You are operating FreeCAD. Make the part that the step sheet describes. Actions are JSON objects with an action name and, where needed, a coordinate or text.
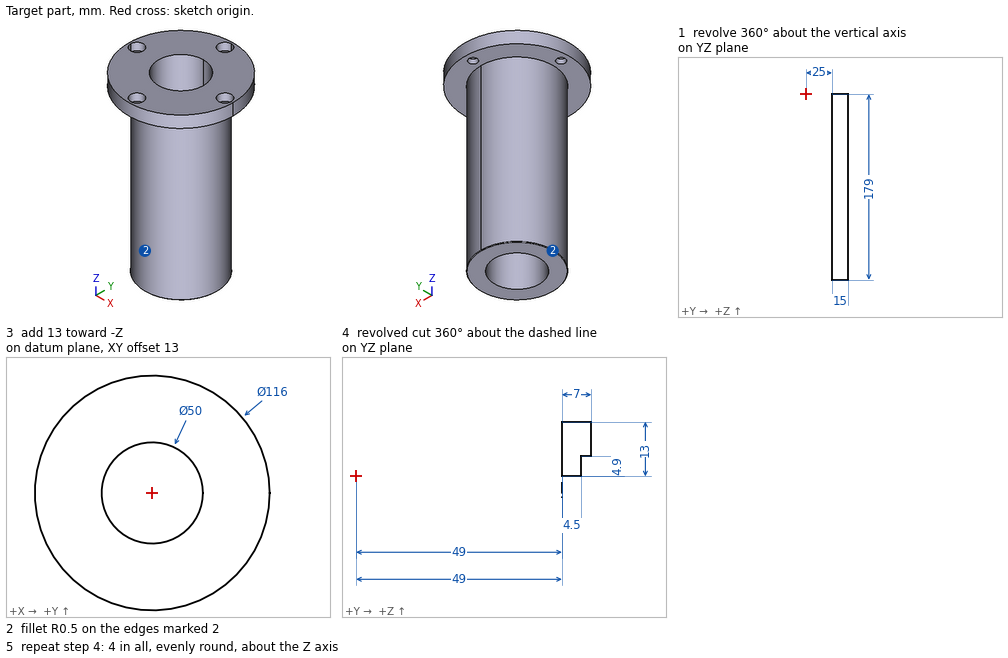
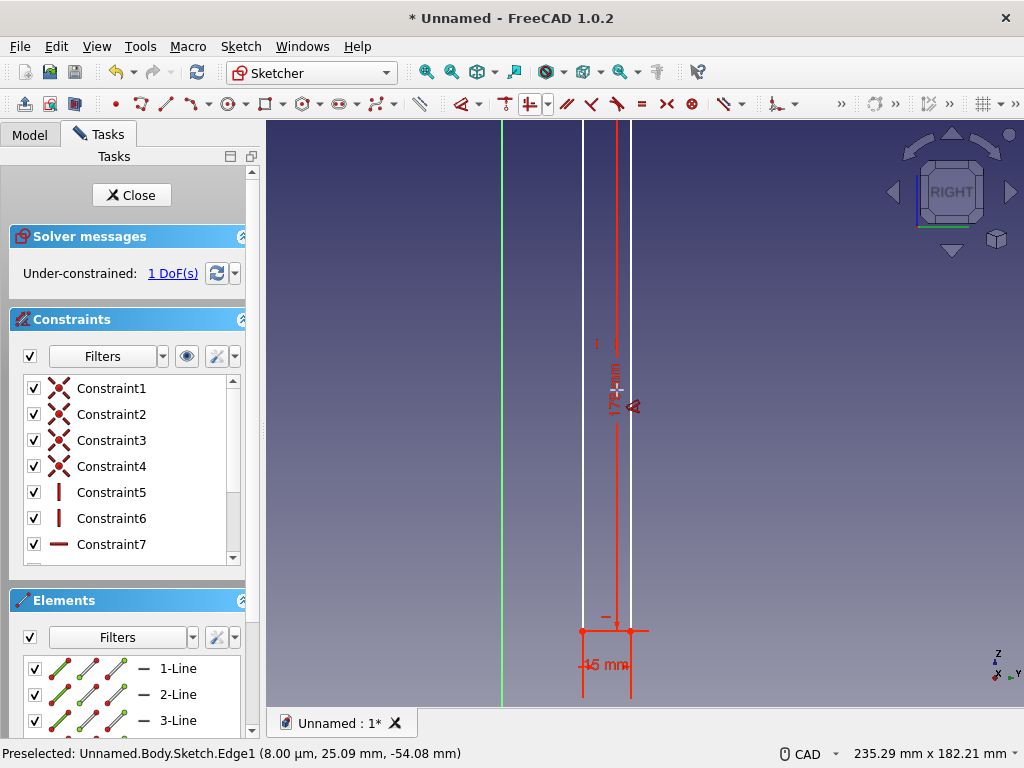
{"action": "scroll", "coordinate": [598, 557], "scroll_direction": "down", "scroll_amount": 2}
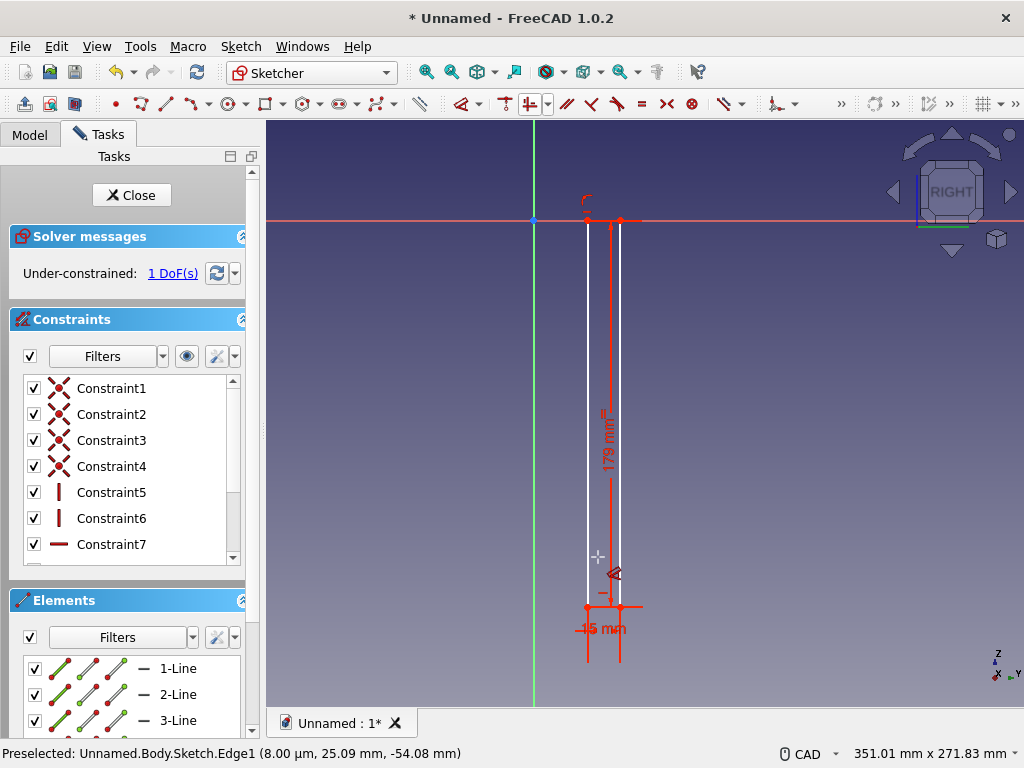
{"action": "left_click", "coordinate": [588, 221]}
{"action": "left_click", "coordinate": [561, 187]}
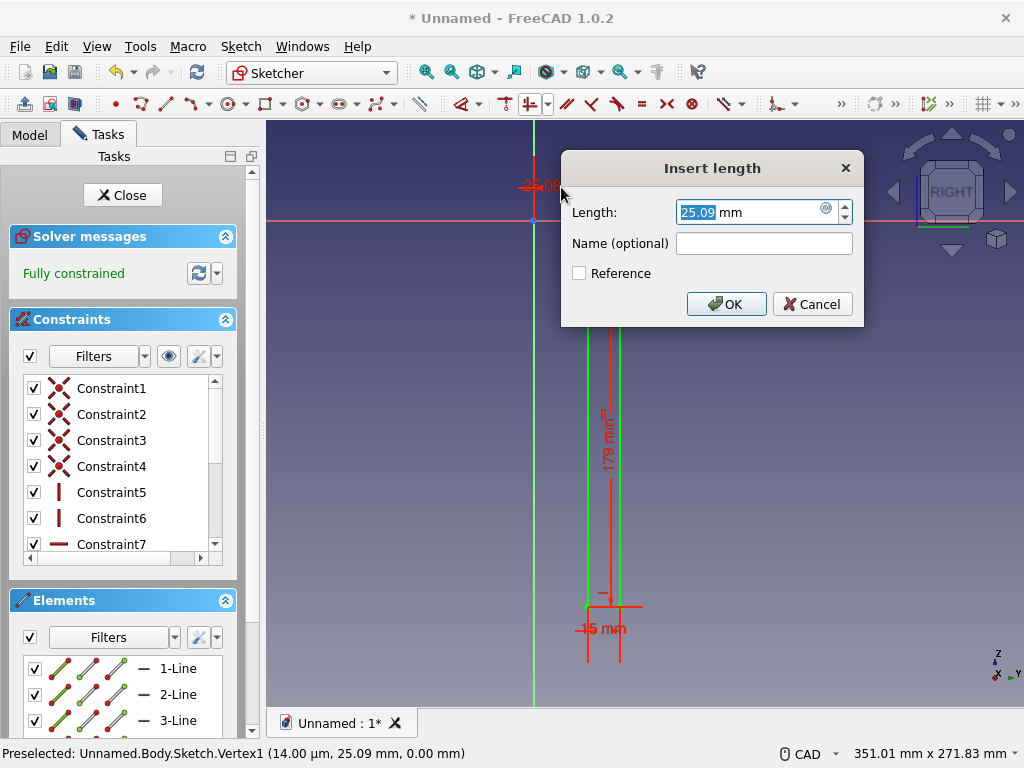
{"action": "type", "text": "25"}
{"action": "key", "text": "Return"}
{"action": "key", "text": "Escape"}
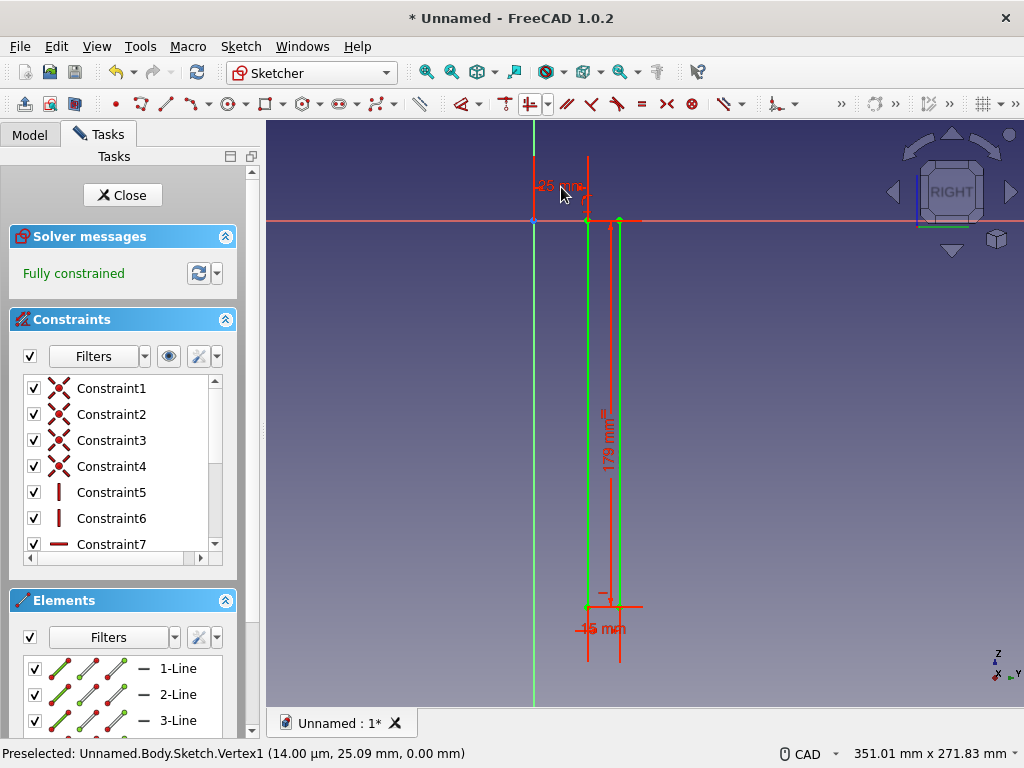
{"action": "left_click", "coordinate": [123, 195]}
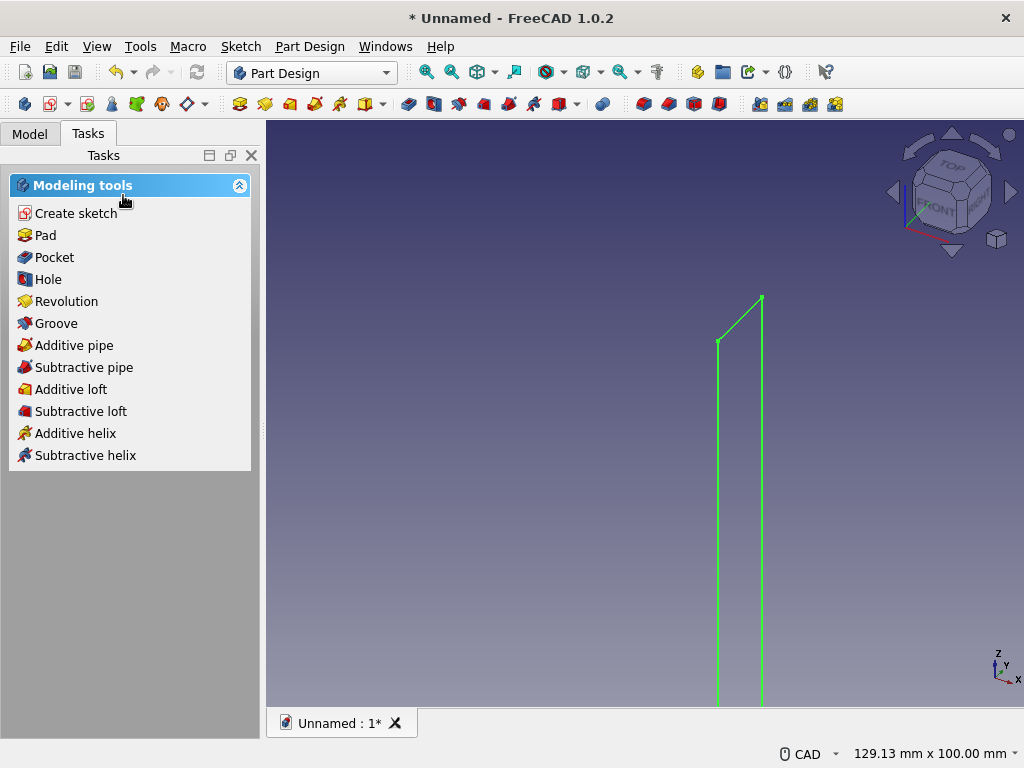
{"action": "left_click", "coordinate": [265, 104]}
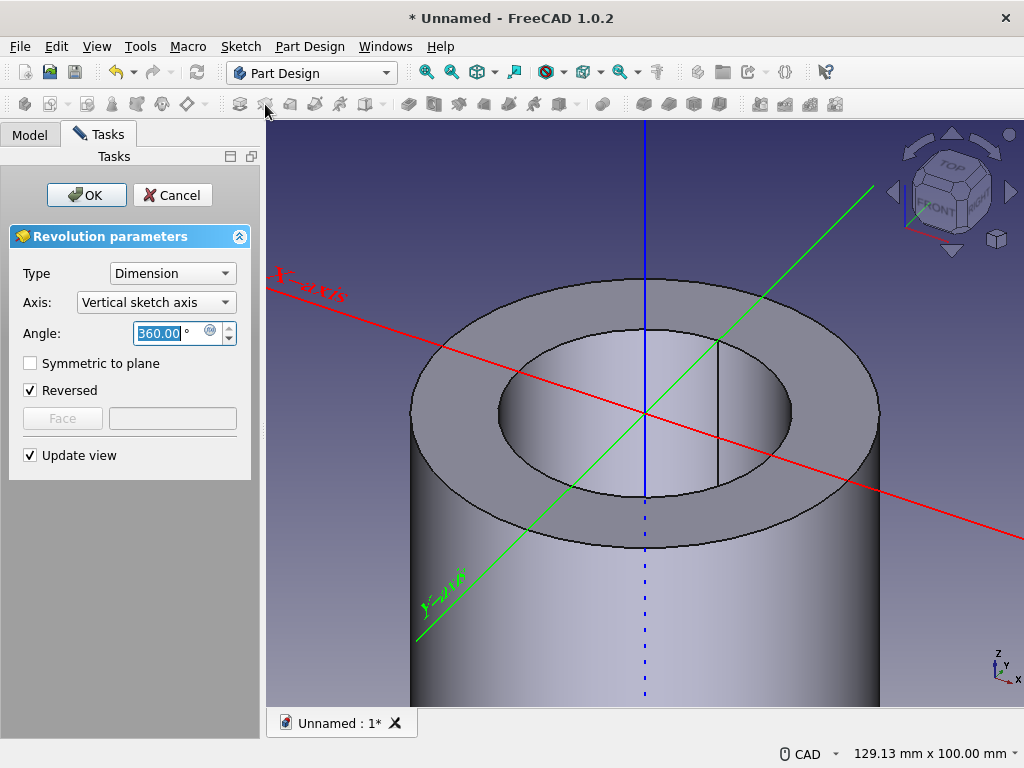
{"action": "left_click", "coordinate": [87, 195]}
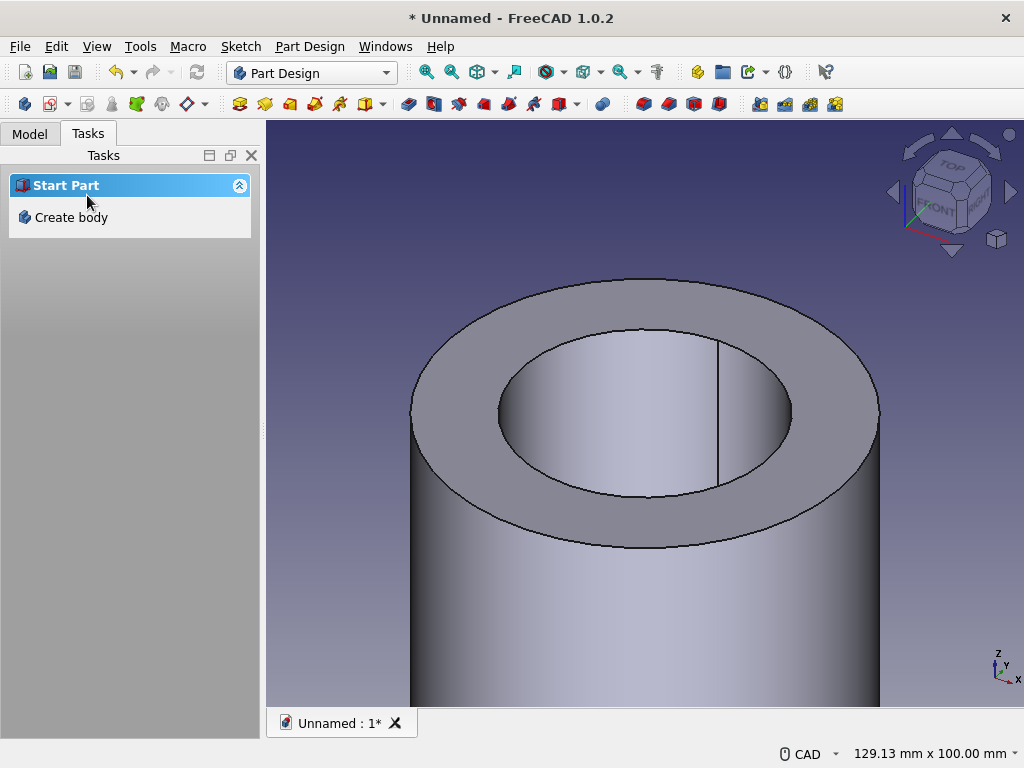
{"action": "left_click", "coordinate": [427, 72]}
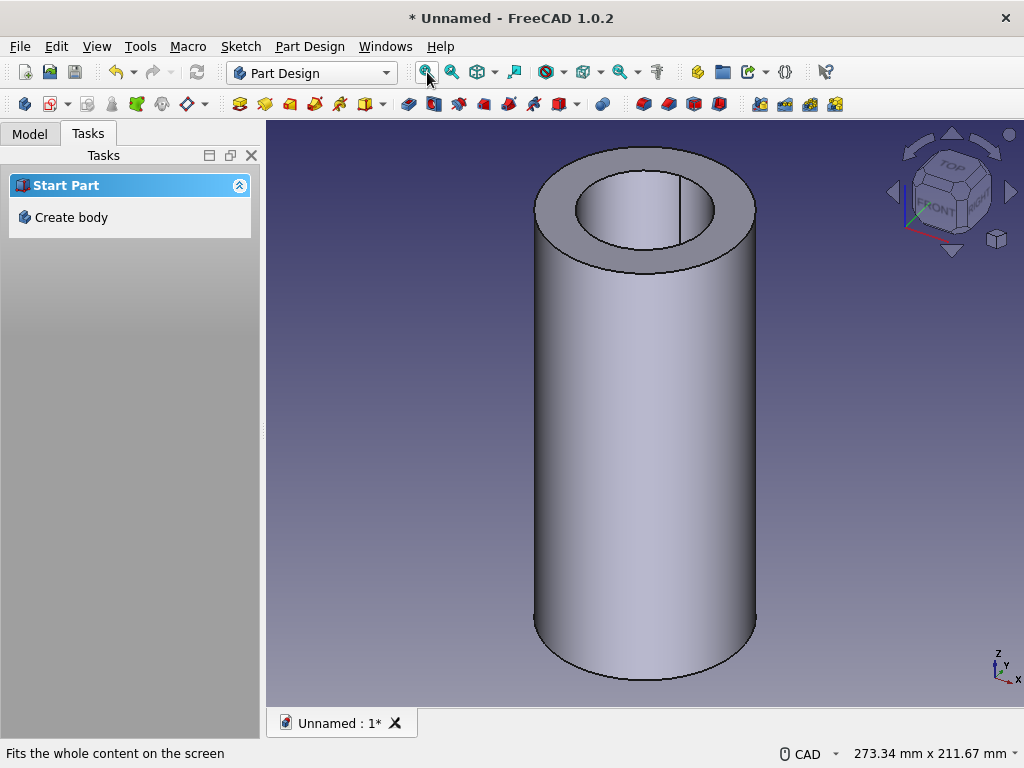
{"action": "key", "text": "0"}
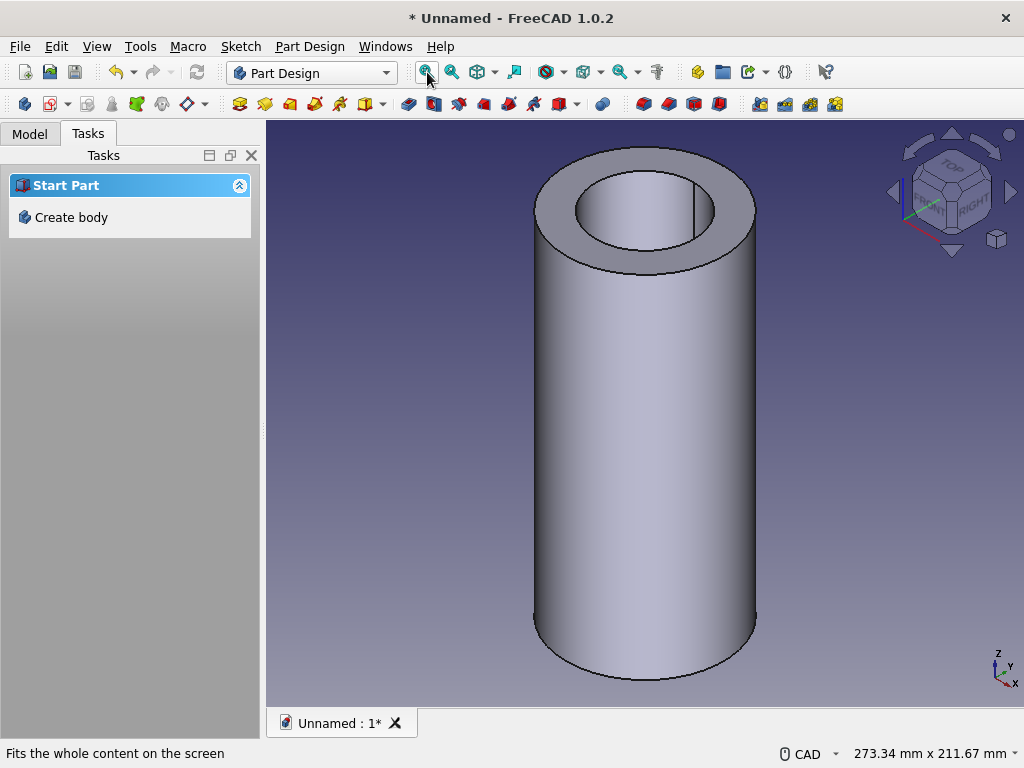
{"action": "left_click", "coordinate": [427, 72]}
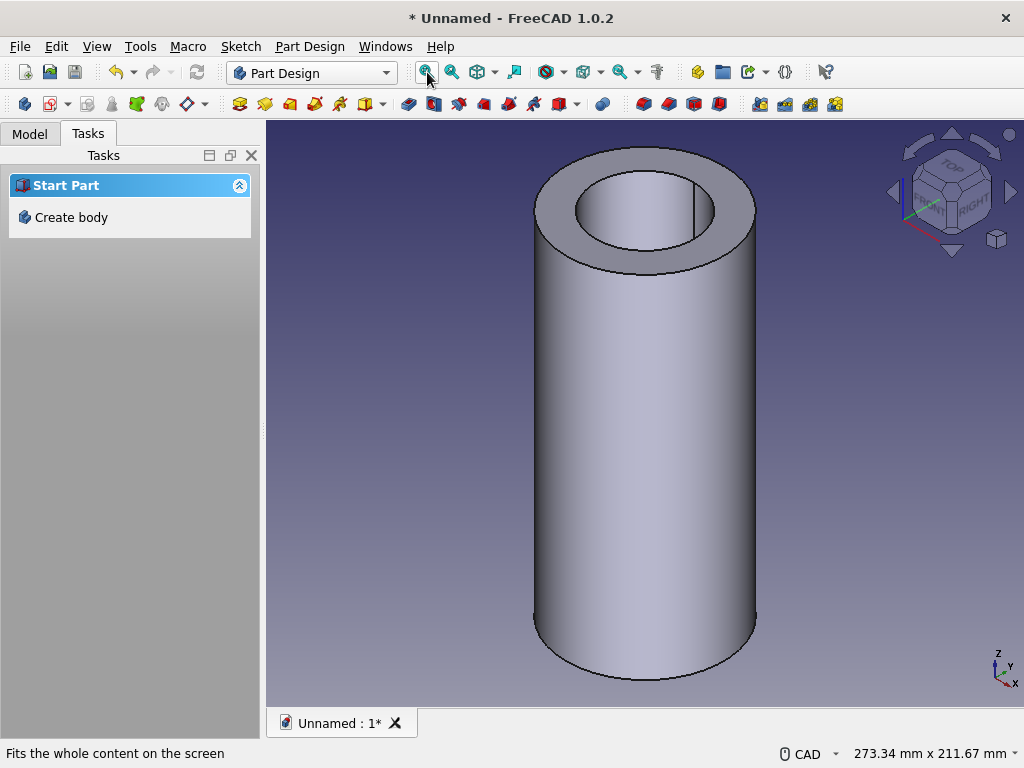
{"action": "key", "text": "2"}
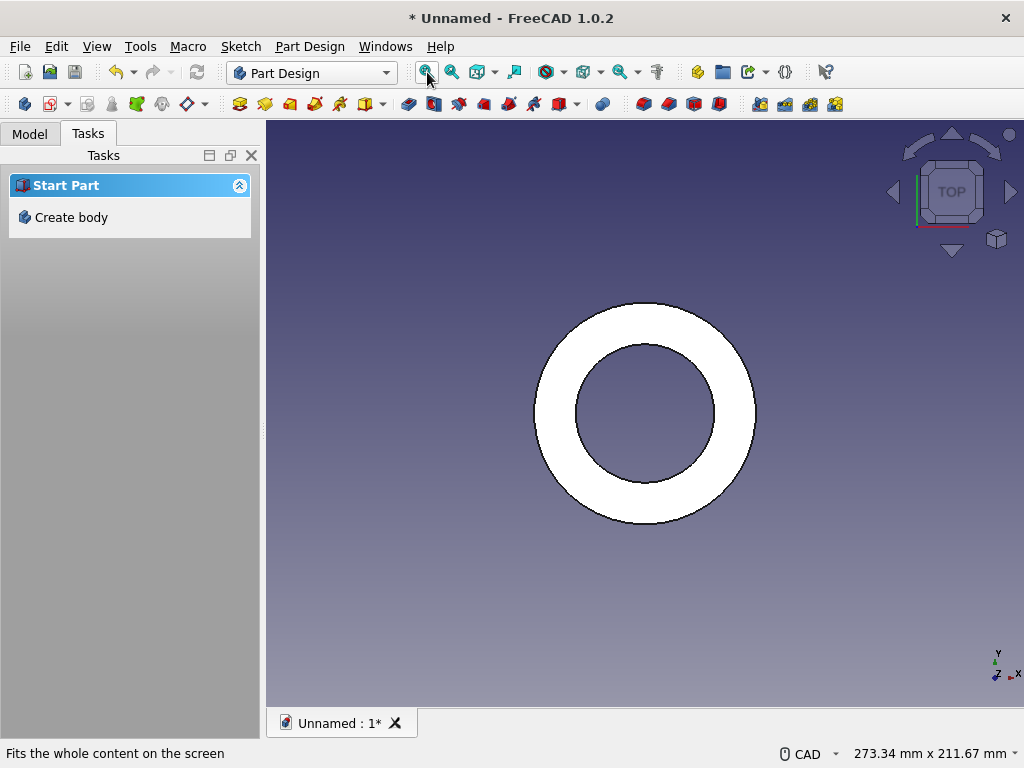
{"action": "left_click", "coordinate": [427, 72]}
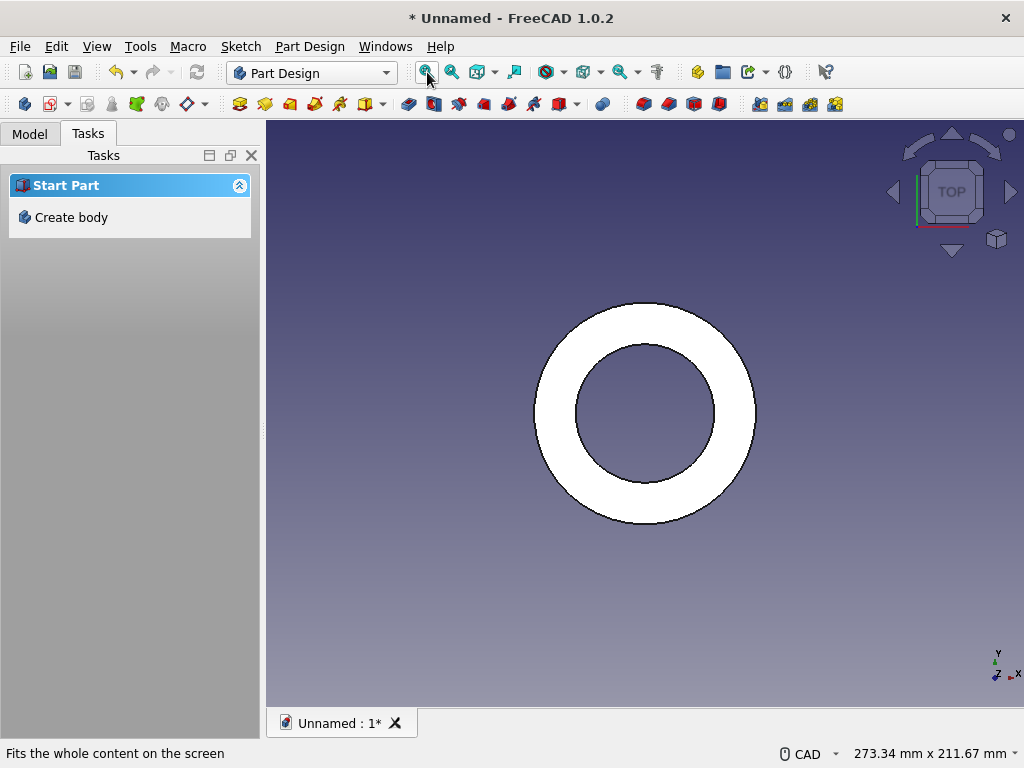
{"action": "key", "text": "1"}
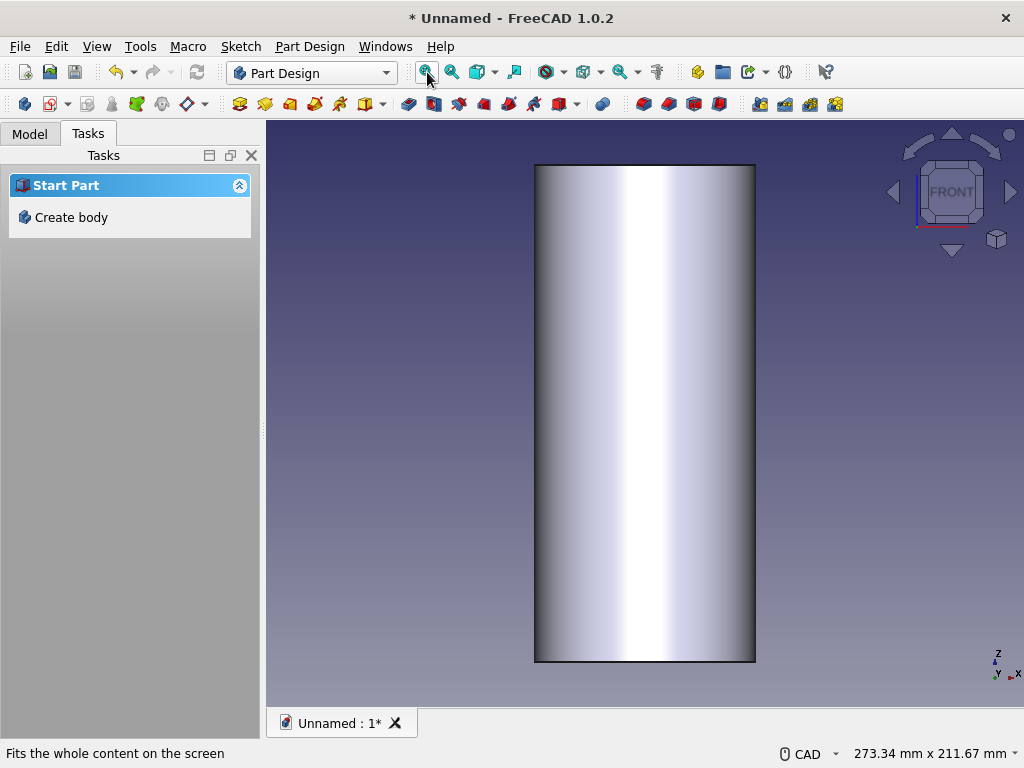
{"action": "left_click", "coordinate": [645, 661]}